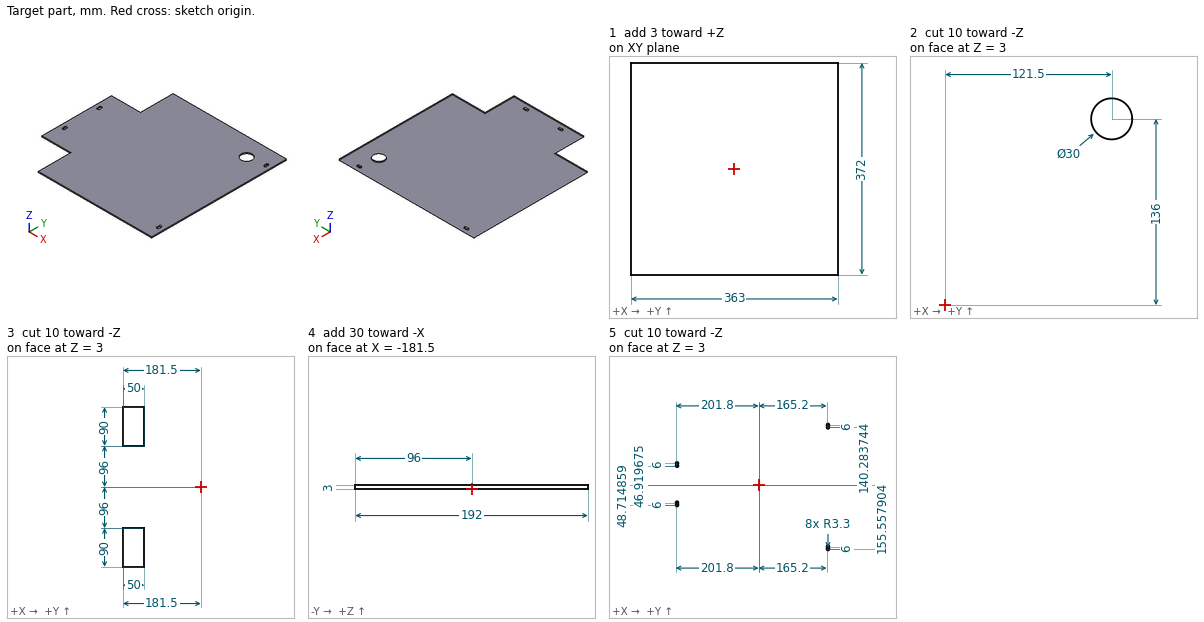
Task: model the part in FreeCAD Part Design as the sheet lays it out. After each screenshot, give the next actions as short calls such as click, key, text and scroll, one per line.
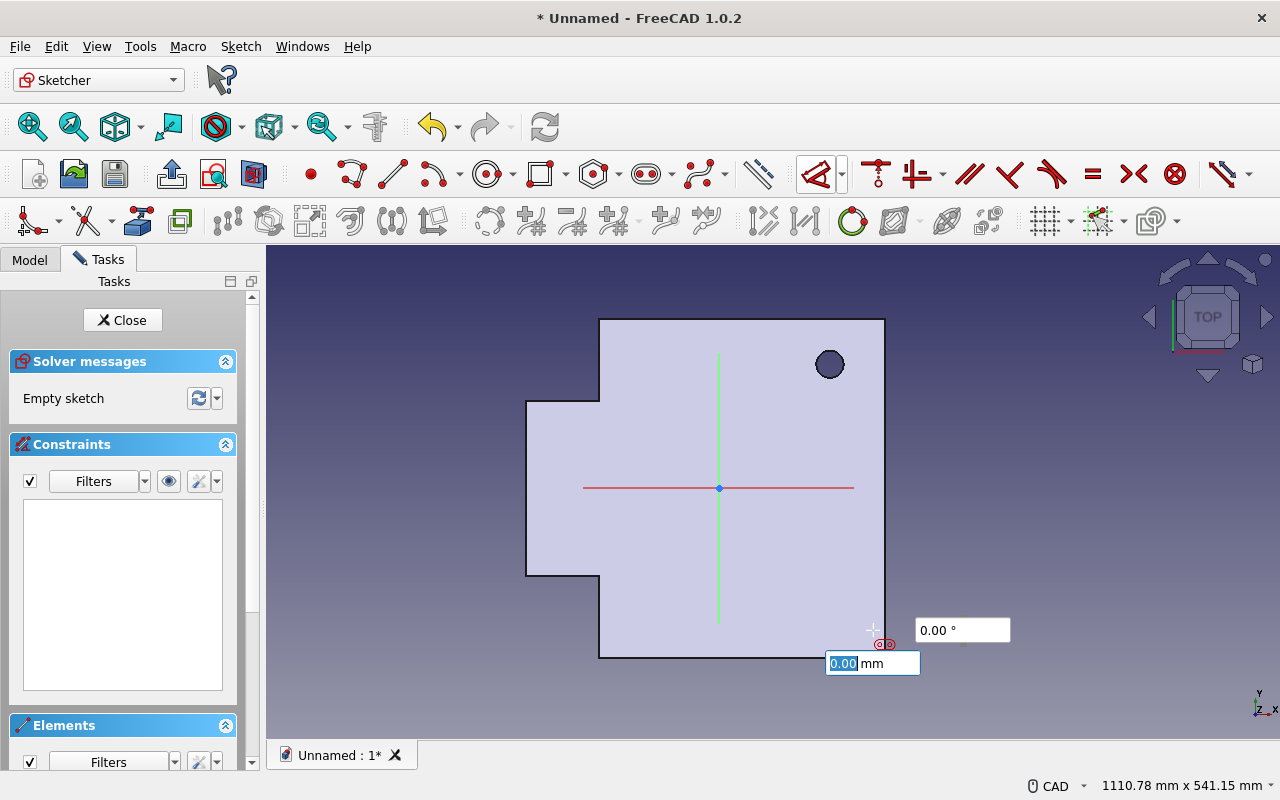
scroll(873, 625, up, 6)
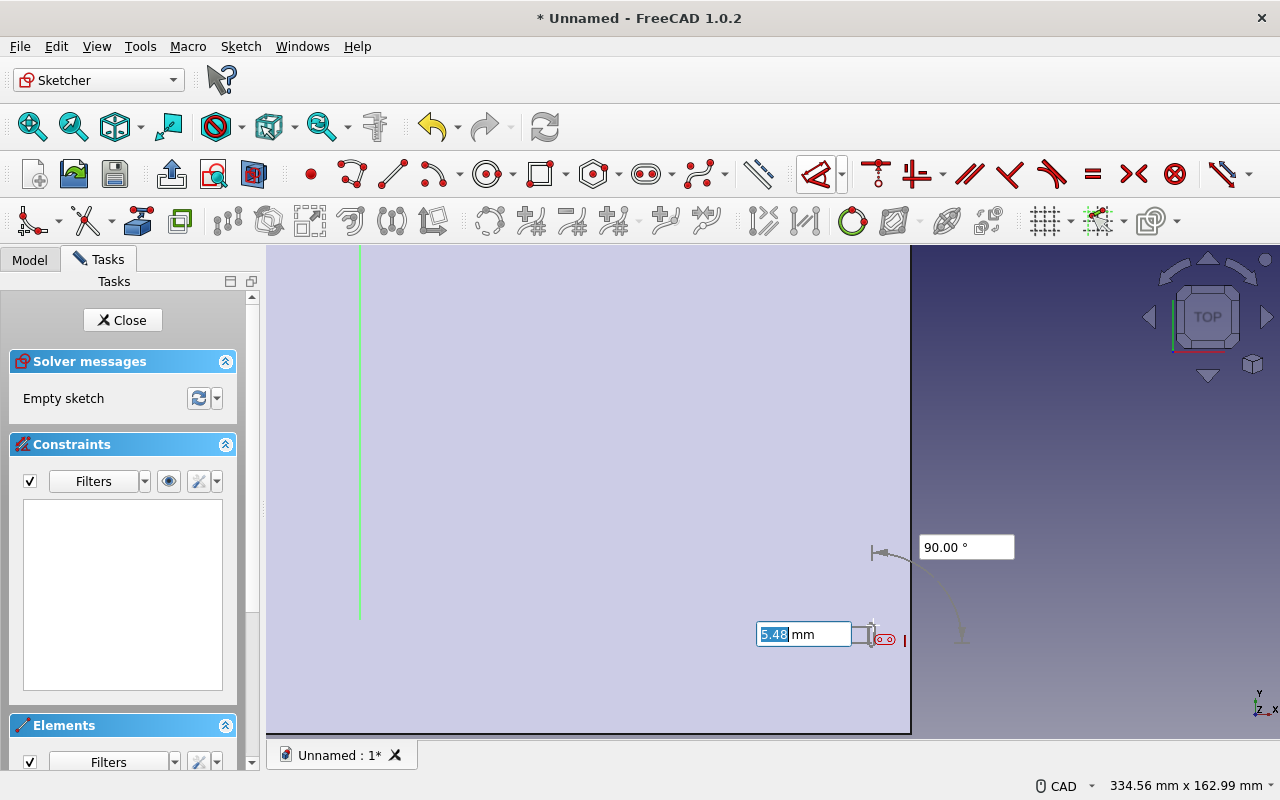
click(872, 623)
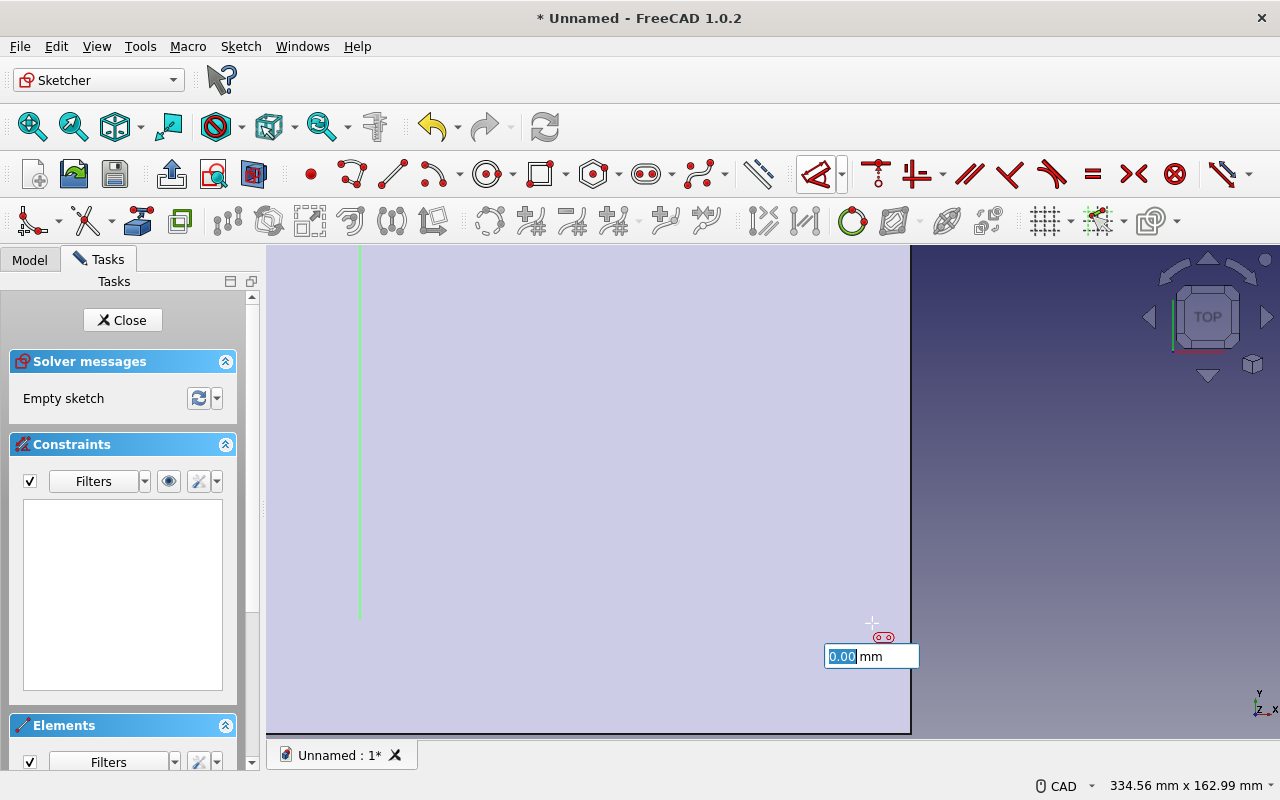
scroll(861, 632, up, 3)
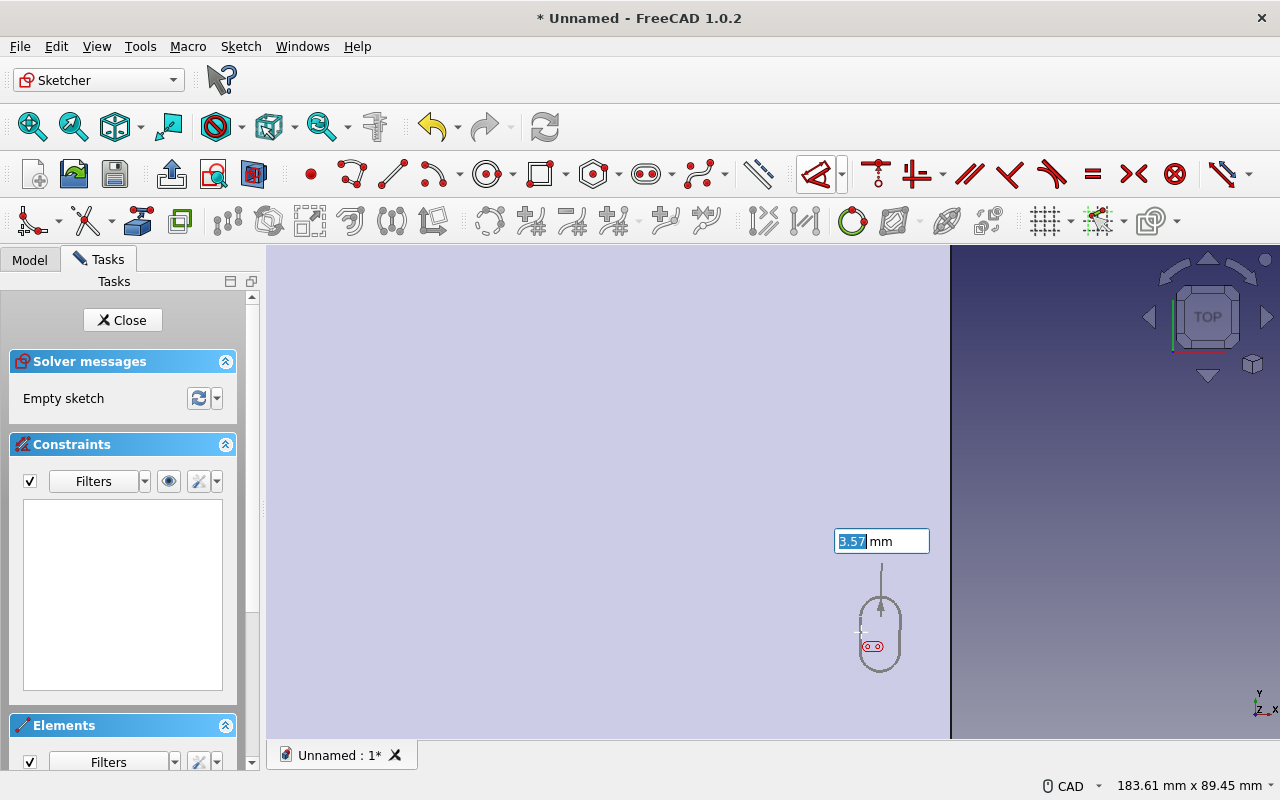
click(861, 632)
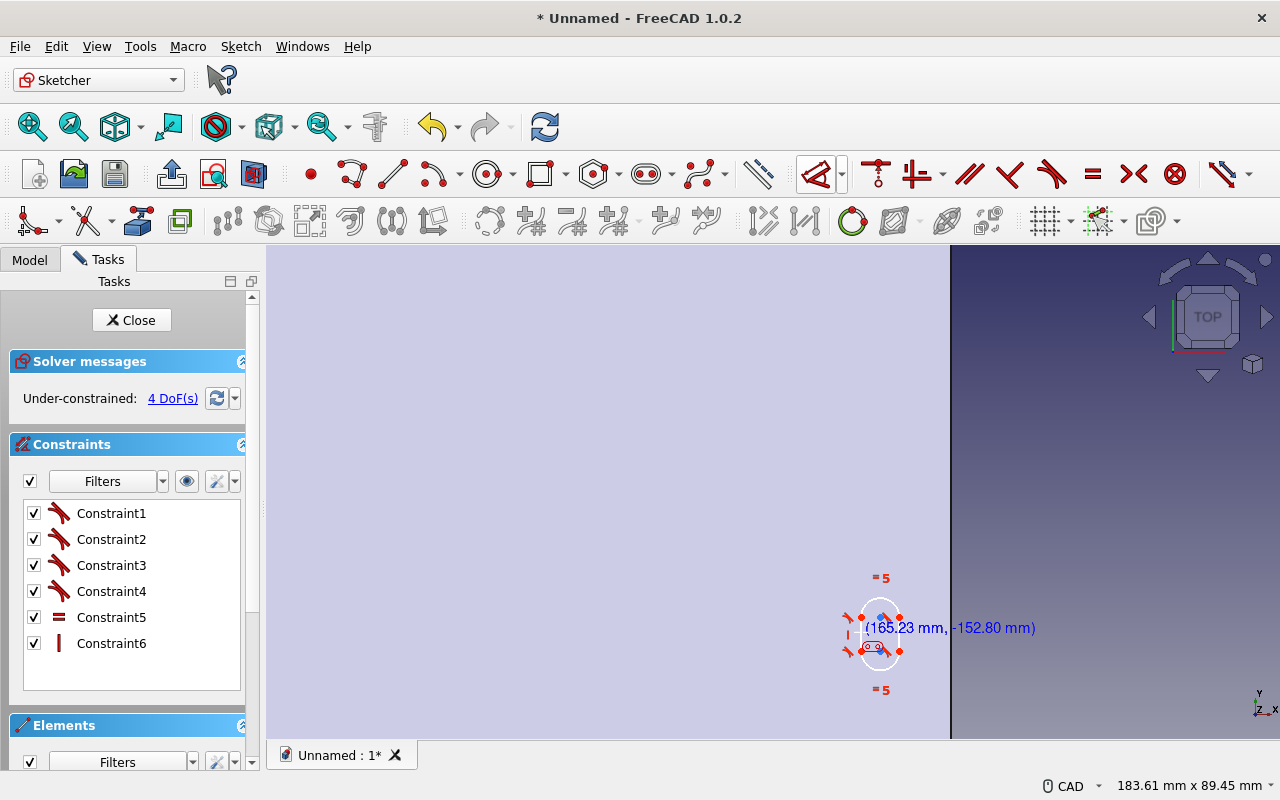
scroll(871, 626, down, 9)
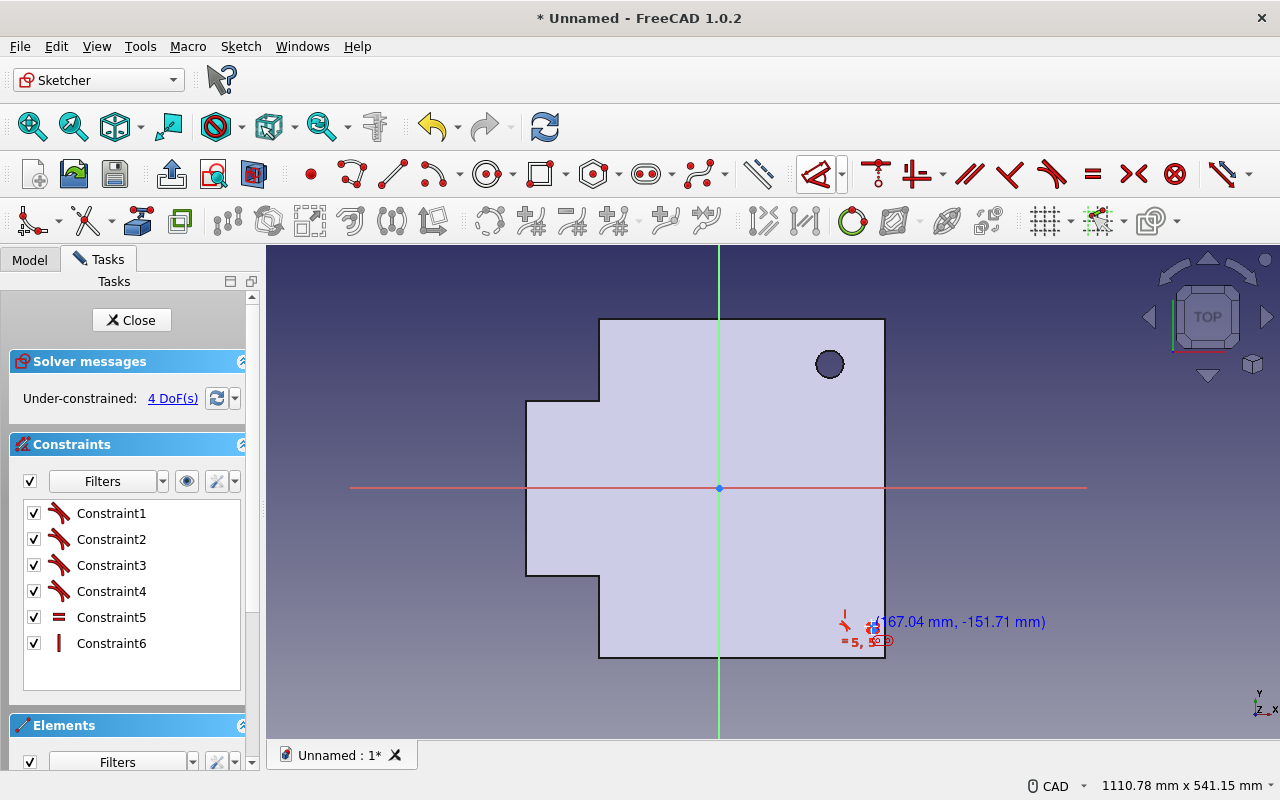
scroll(873, 360, up, 11)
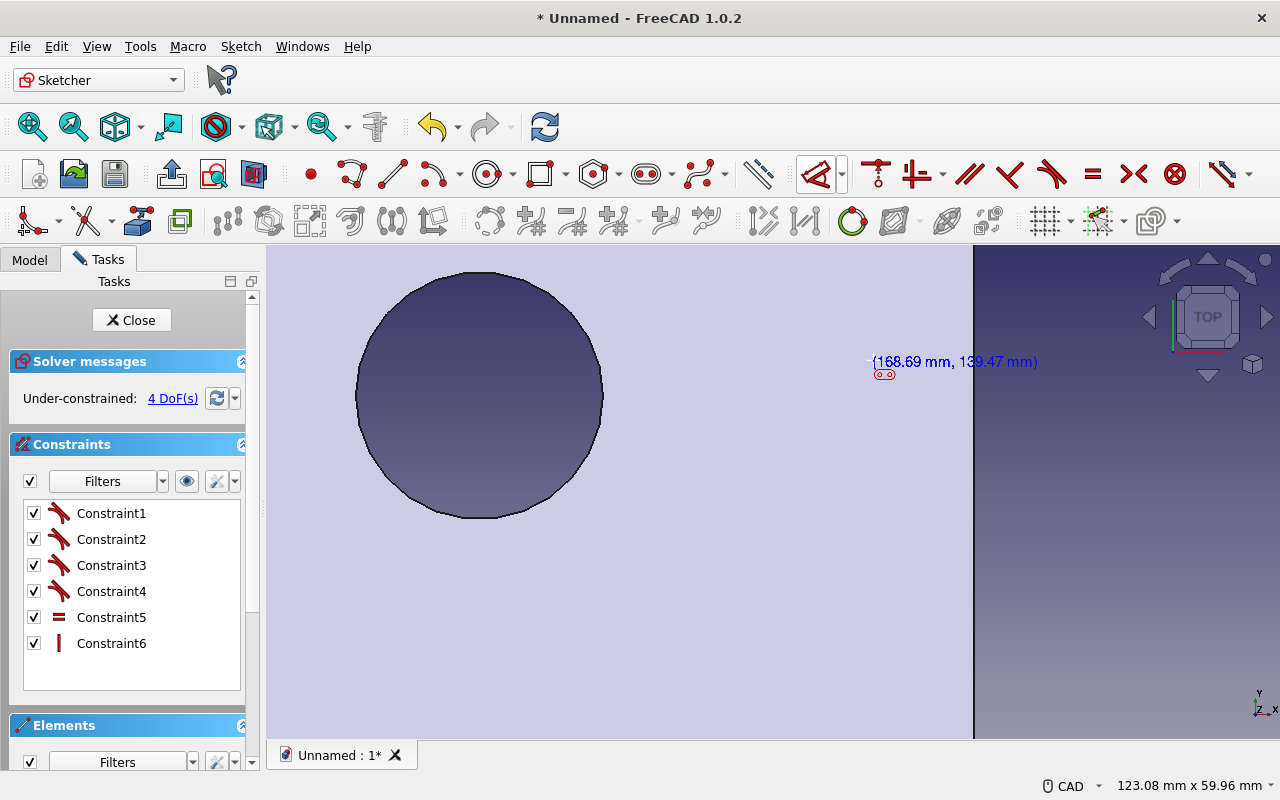
scroll(873, 360, down, 11)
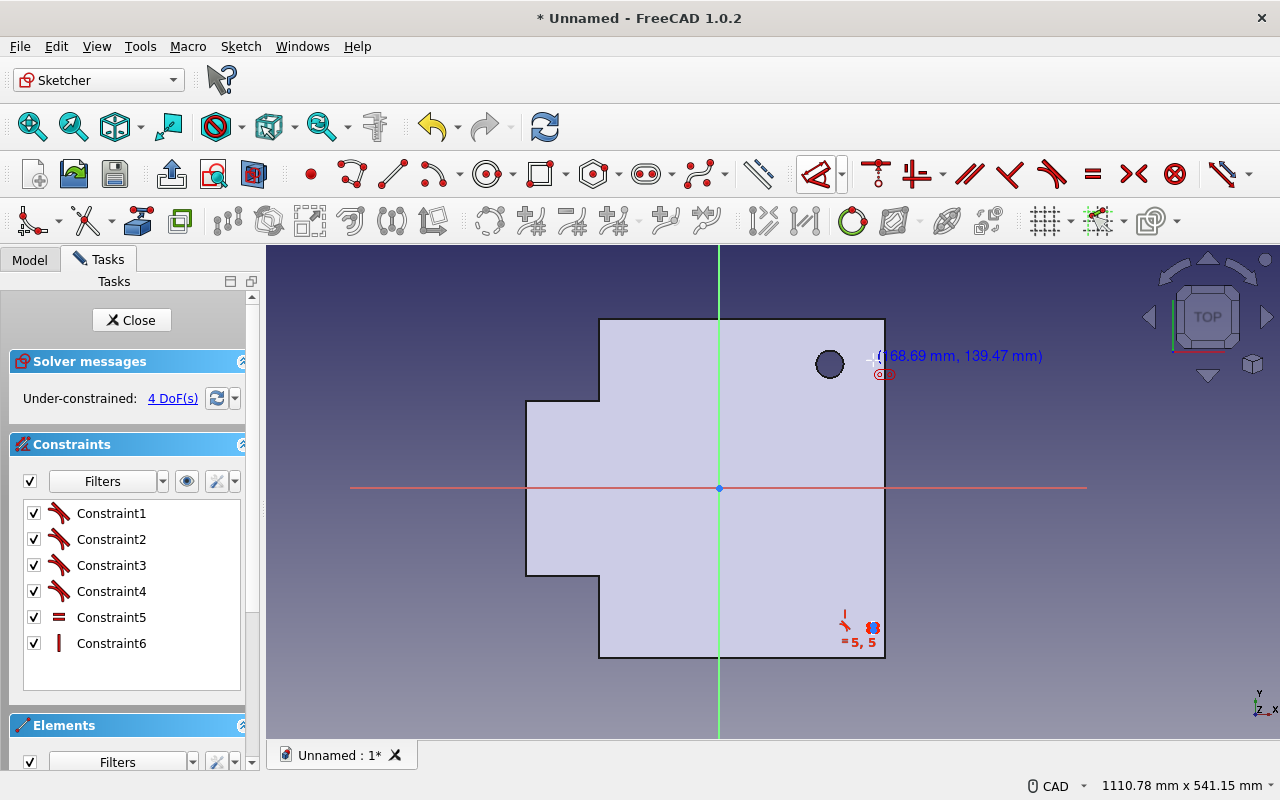
click(873, 360)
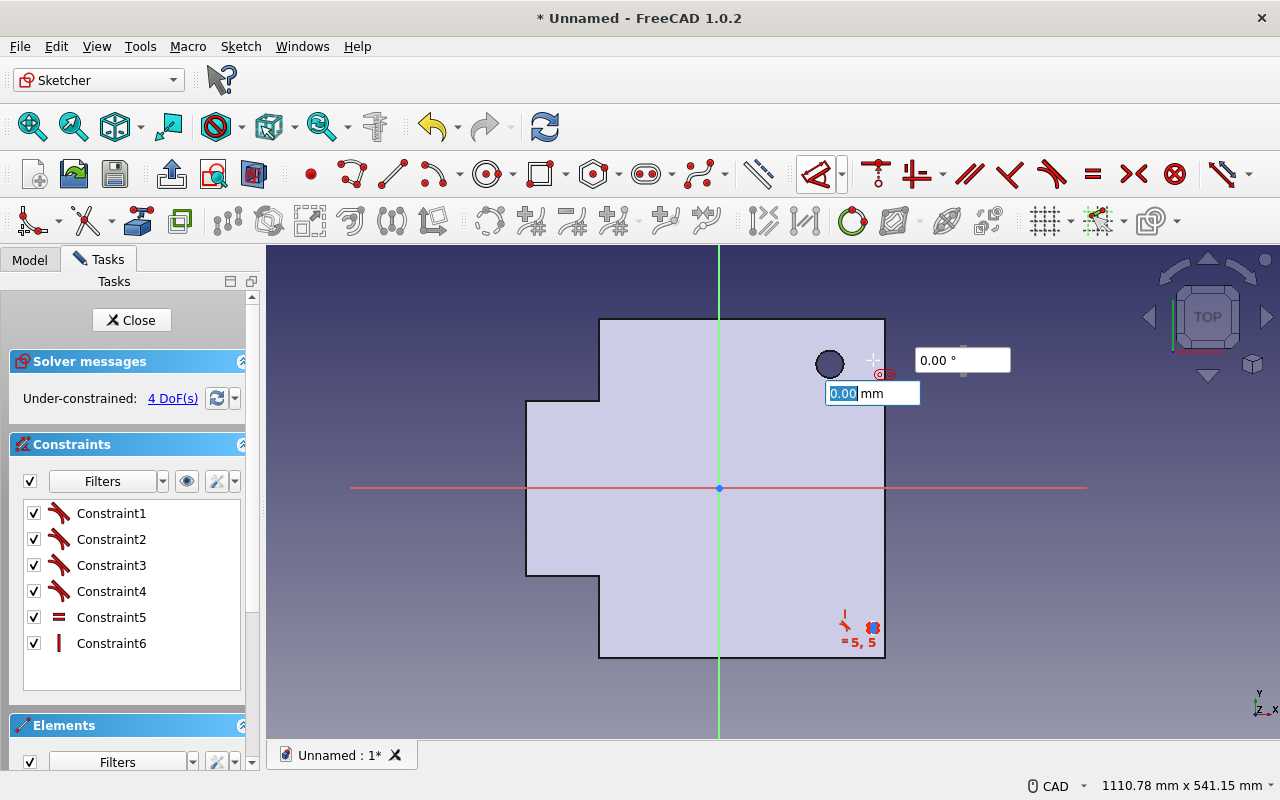
scroll(873, 355, up, 6)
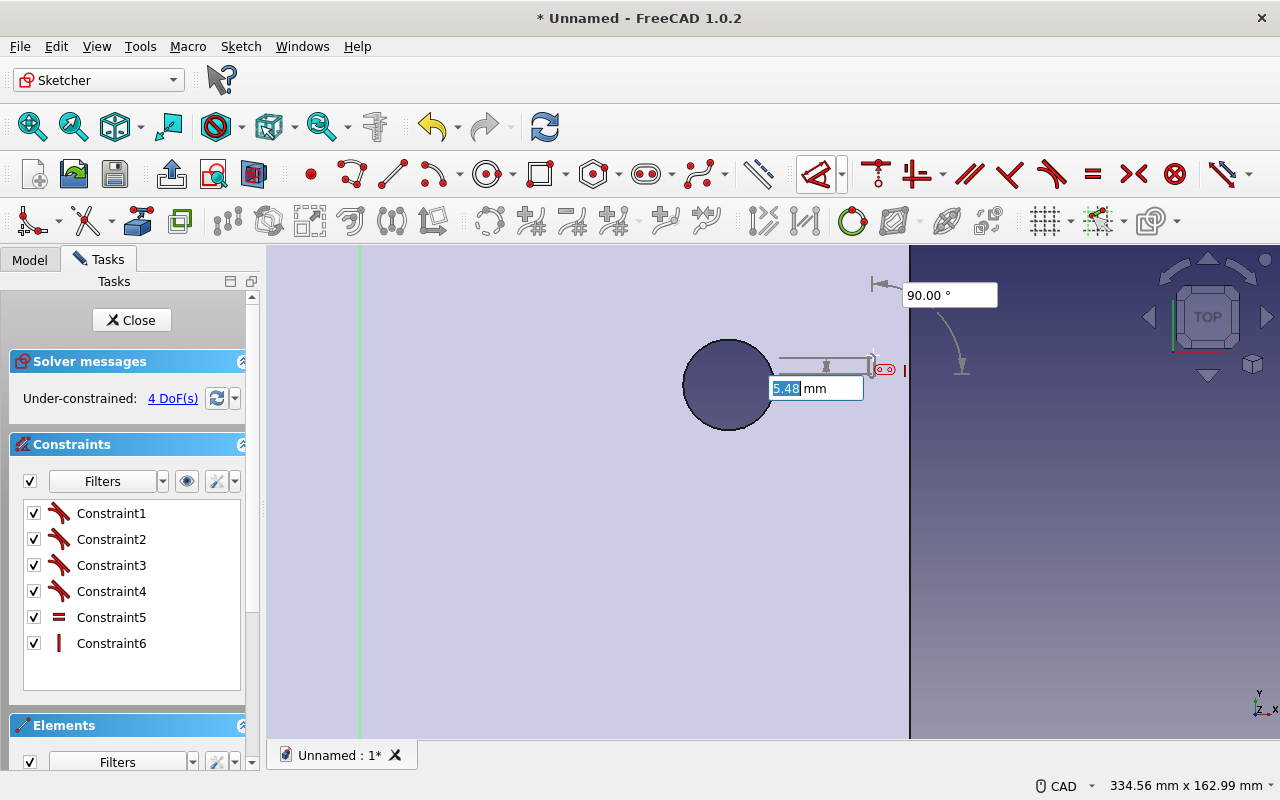
click(872, 354)